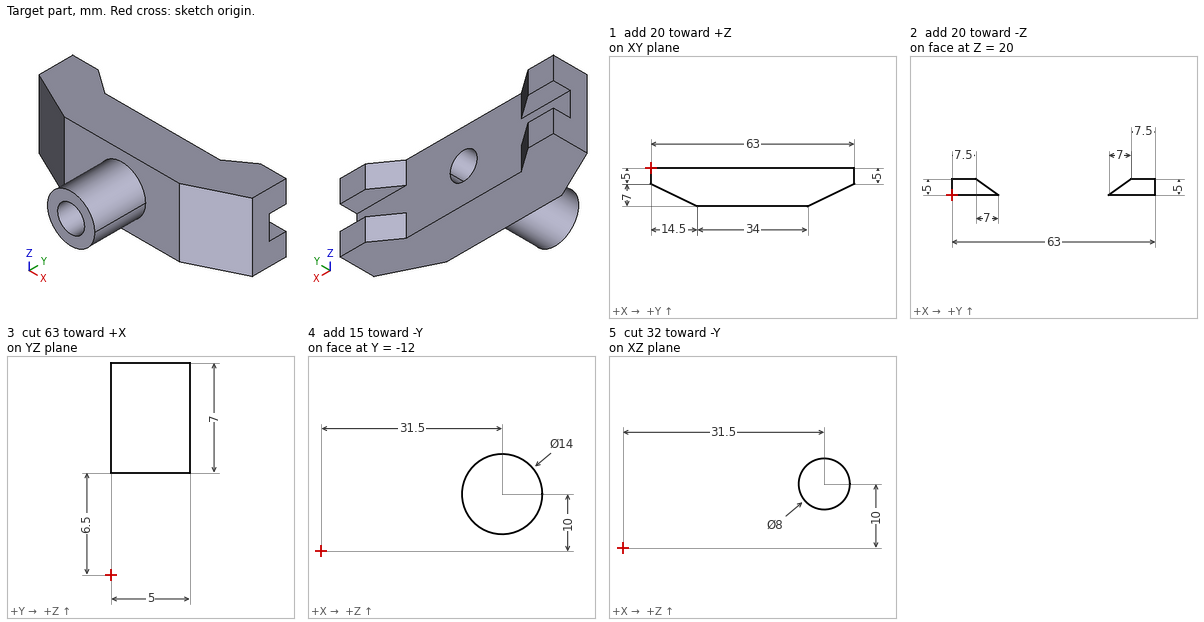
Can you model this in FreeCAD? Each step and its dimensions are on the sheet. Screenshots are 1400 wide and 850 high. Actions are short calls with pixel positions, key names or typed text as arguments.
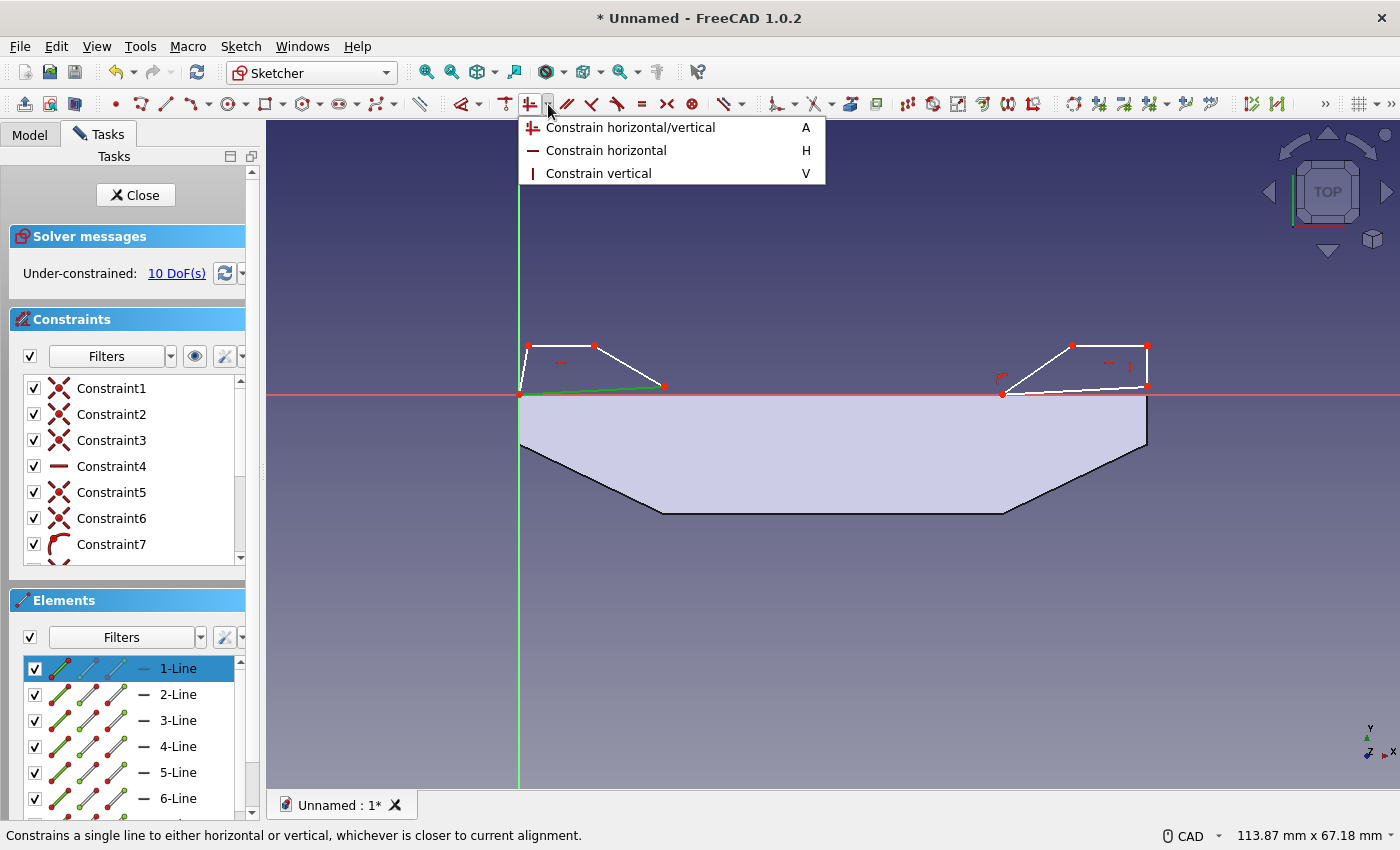
click(672, 150)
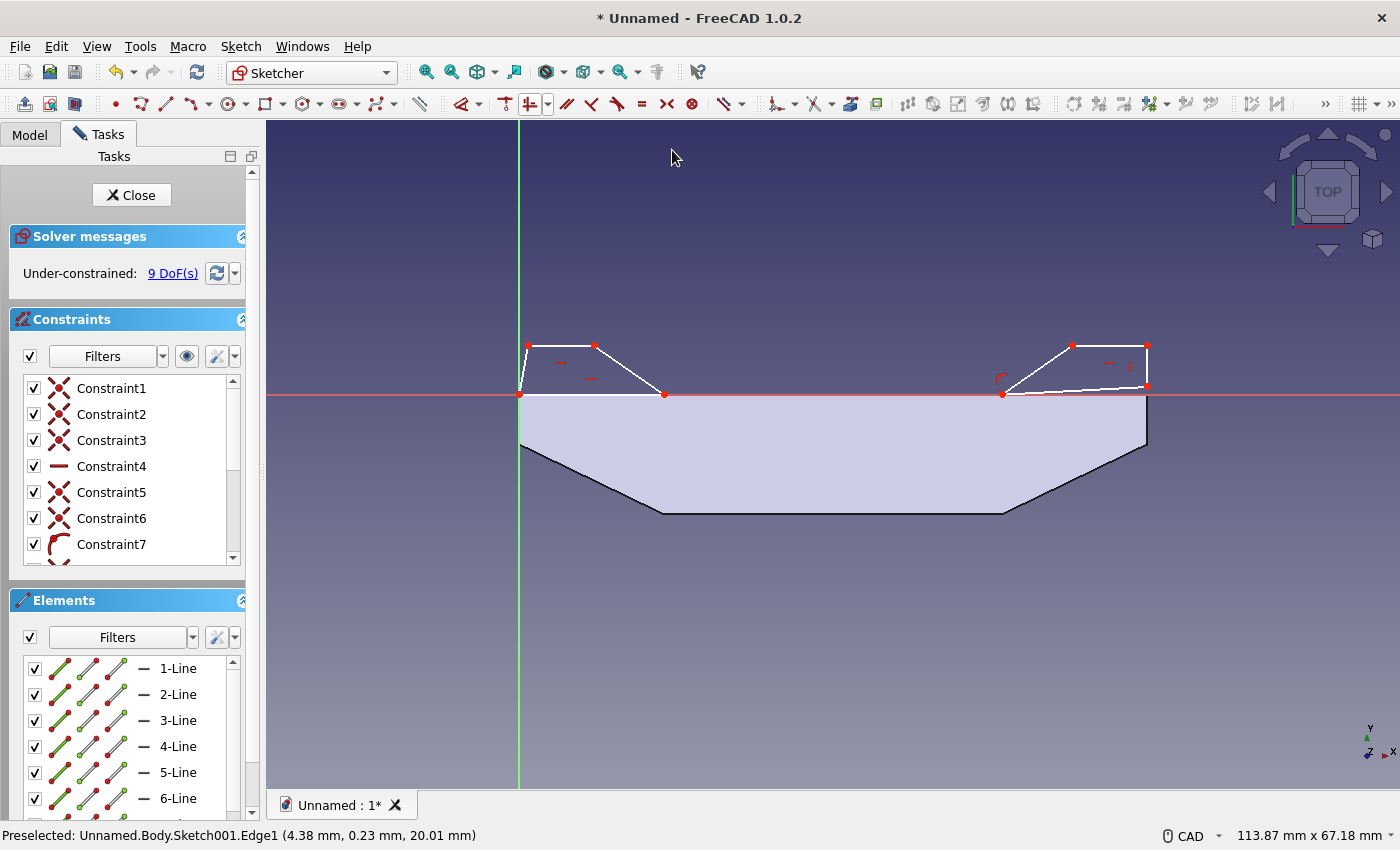
click(522, 380)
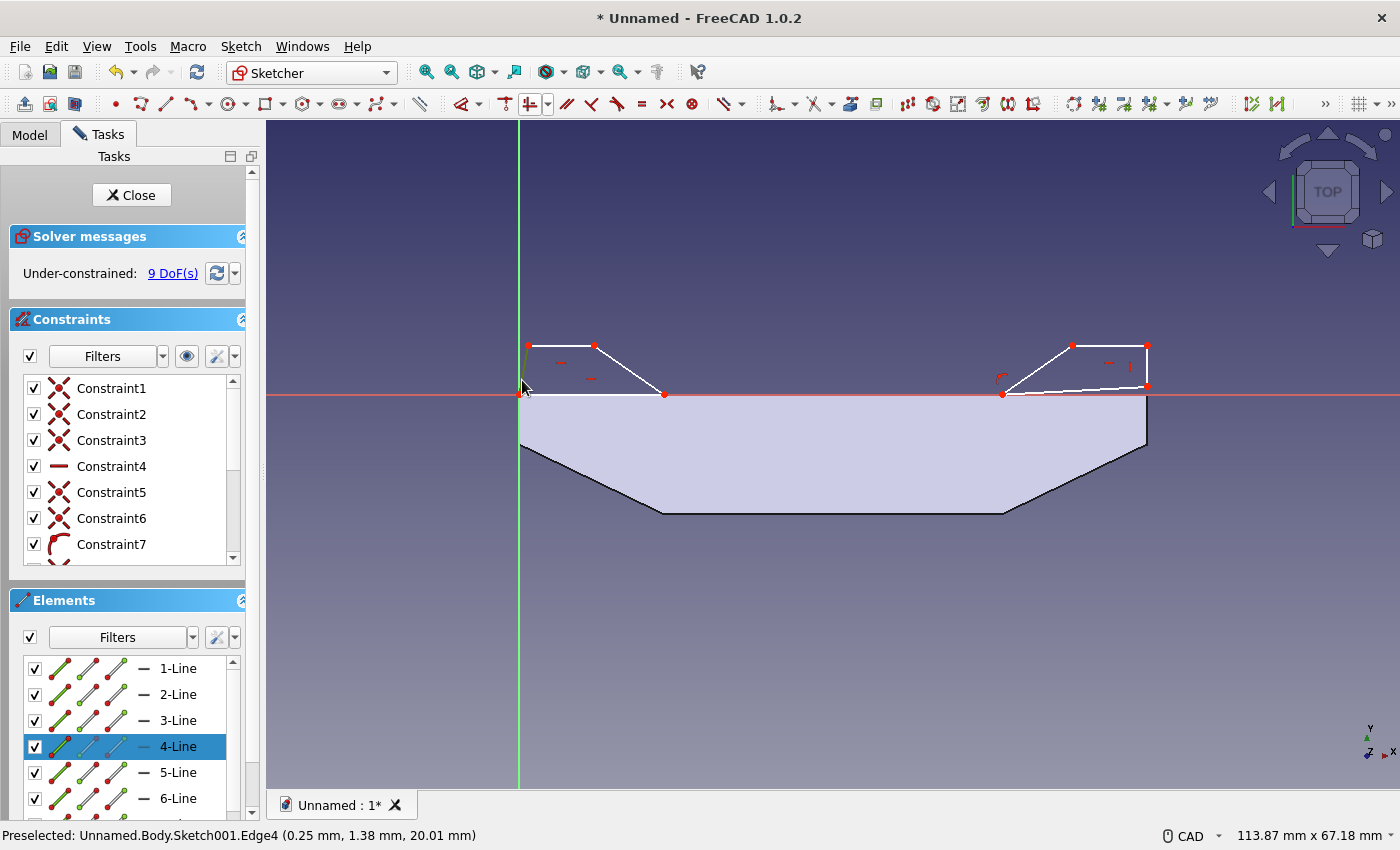
key(v)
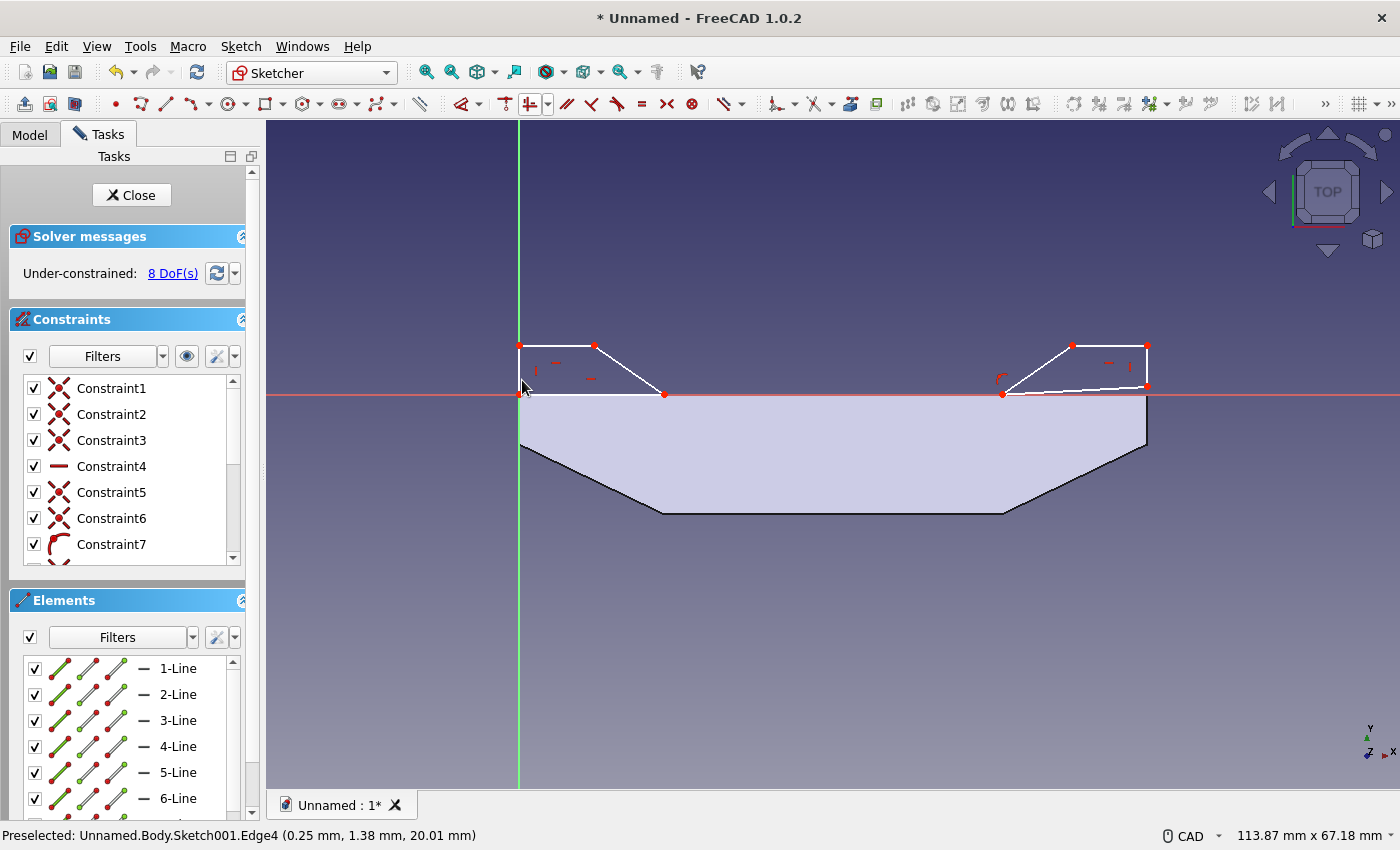
click(1045, 392)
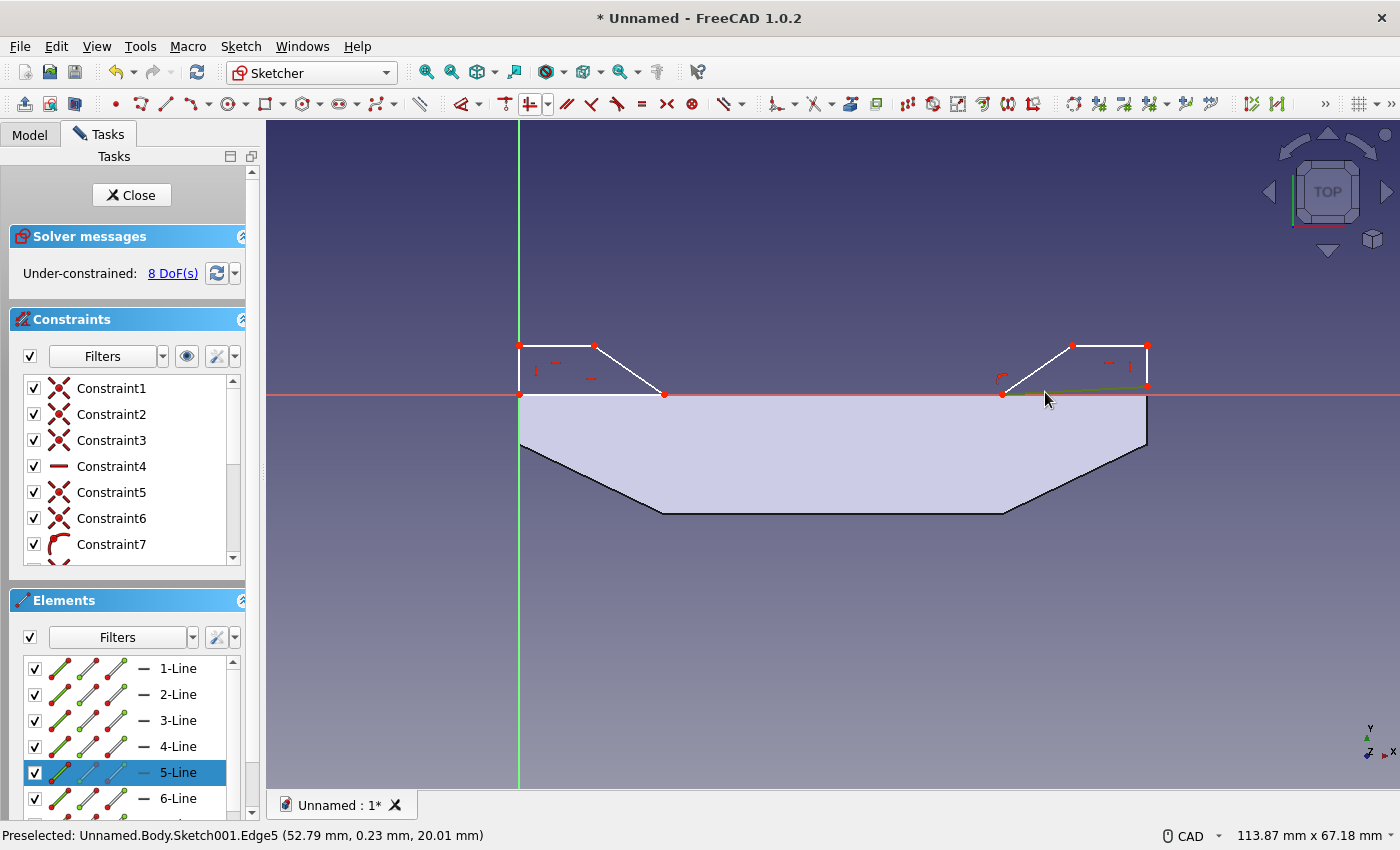
click(548, 104)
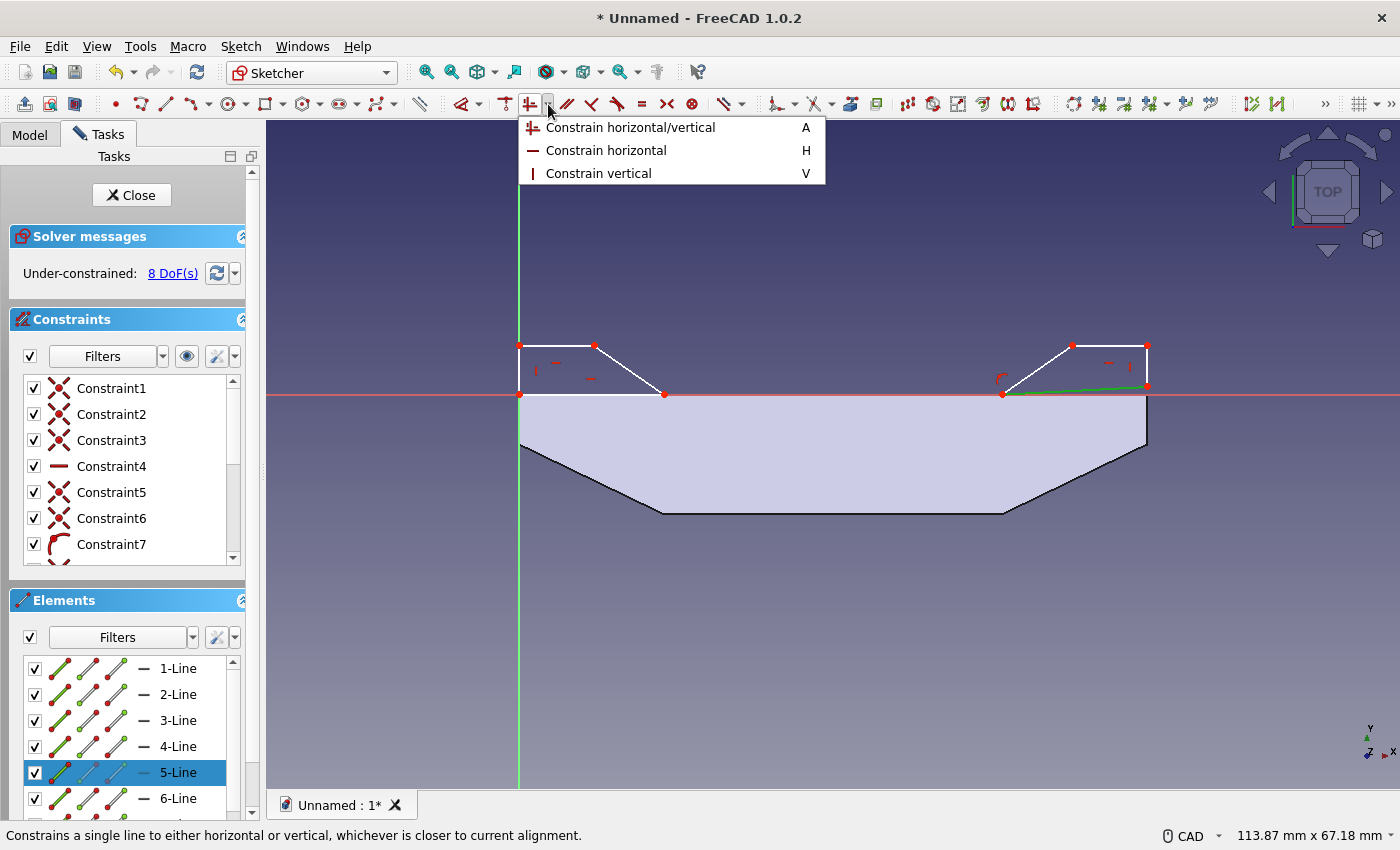
click(672, 150)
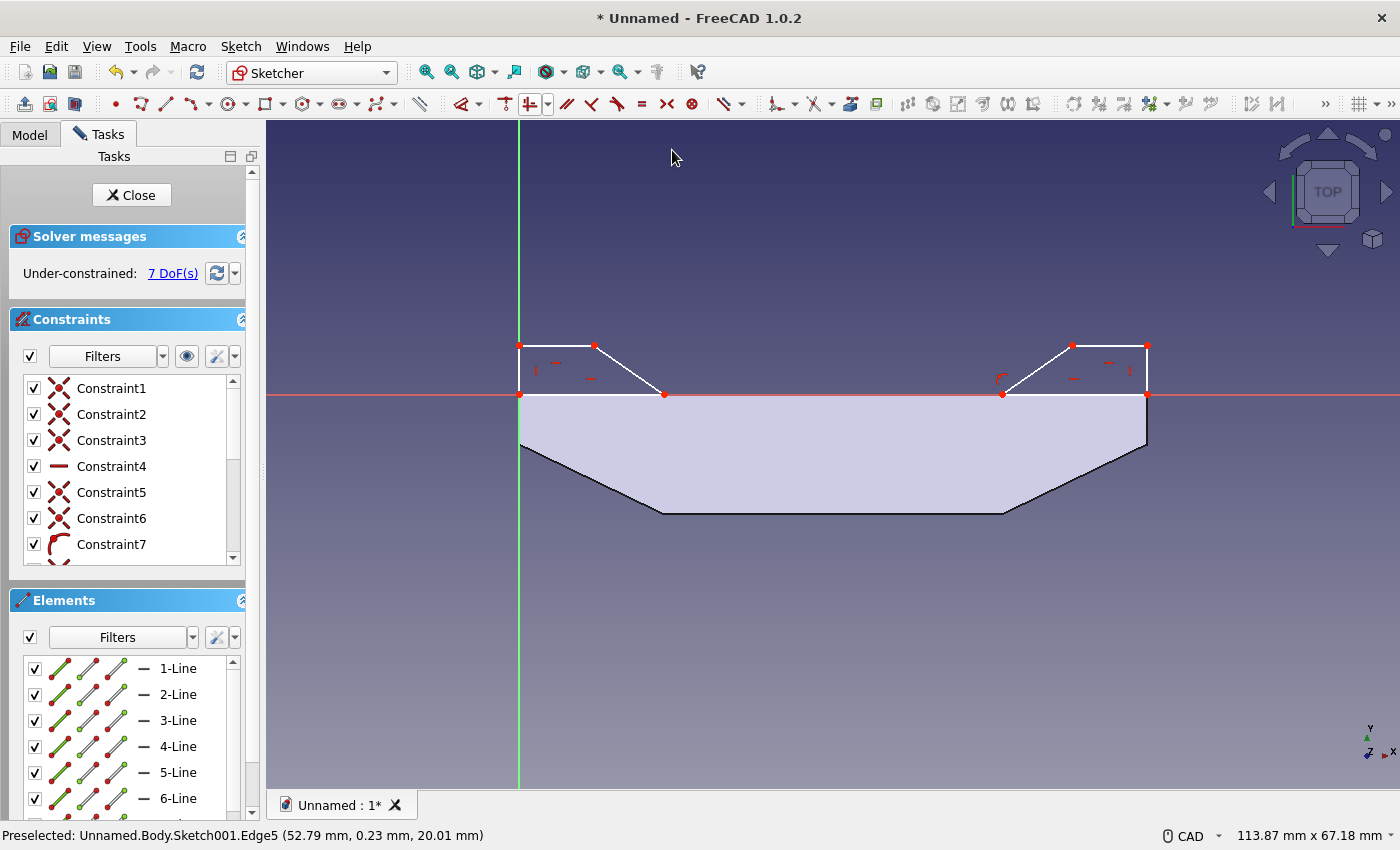
click(460, 104)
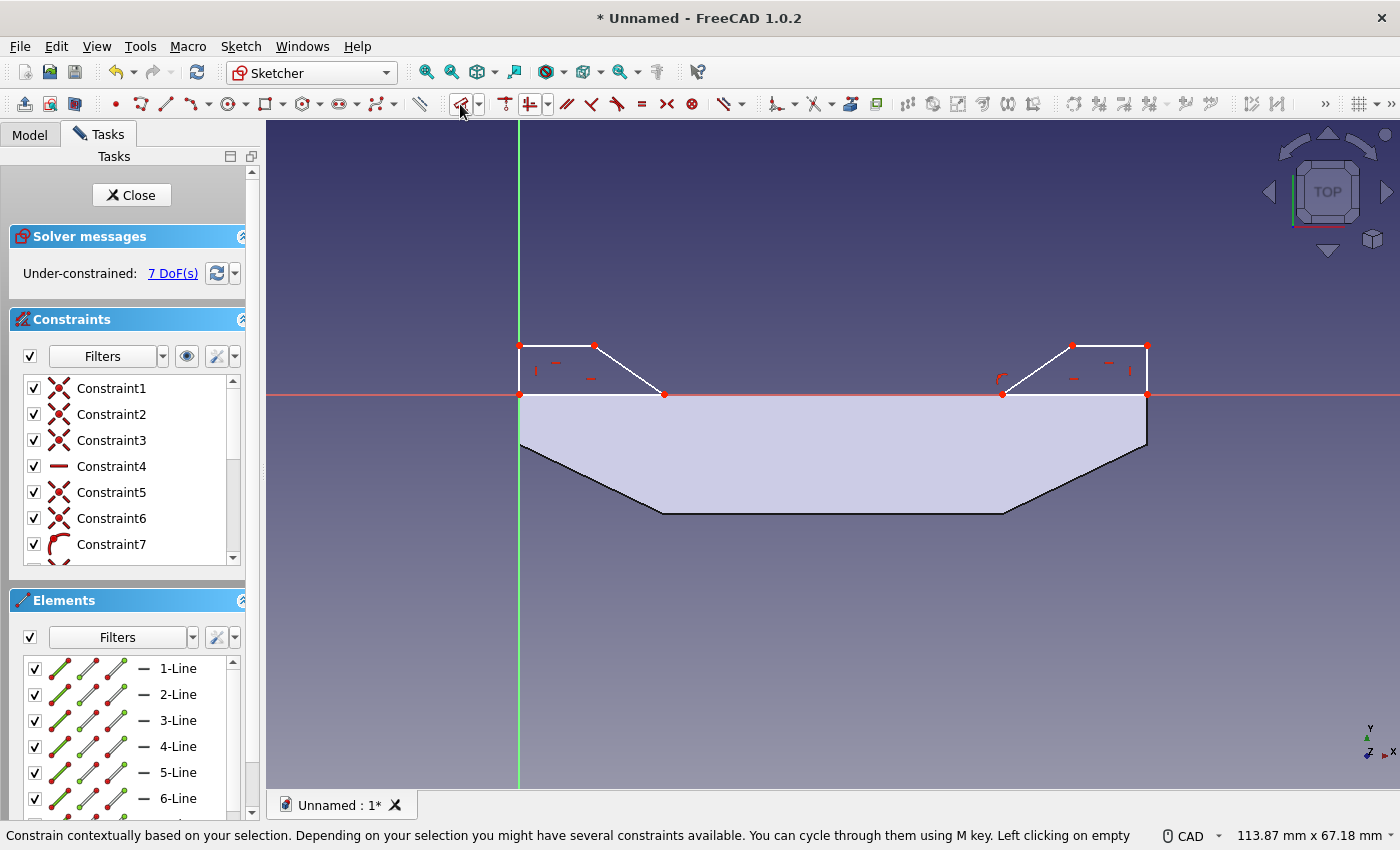
click(519, 361)
click(485, 370)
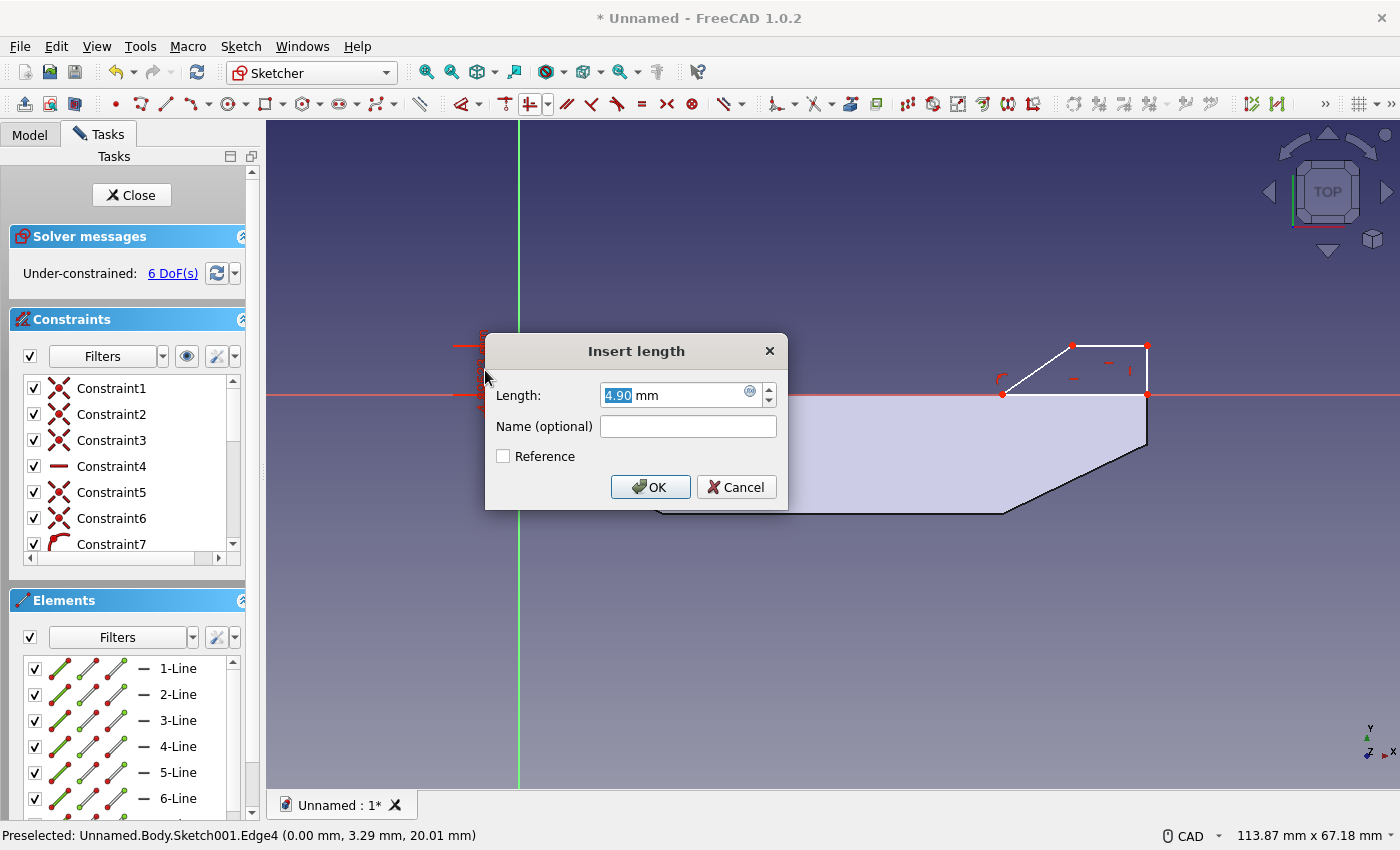
text(5)
key(Return)